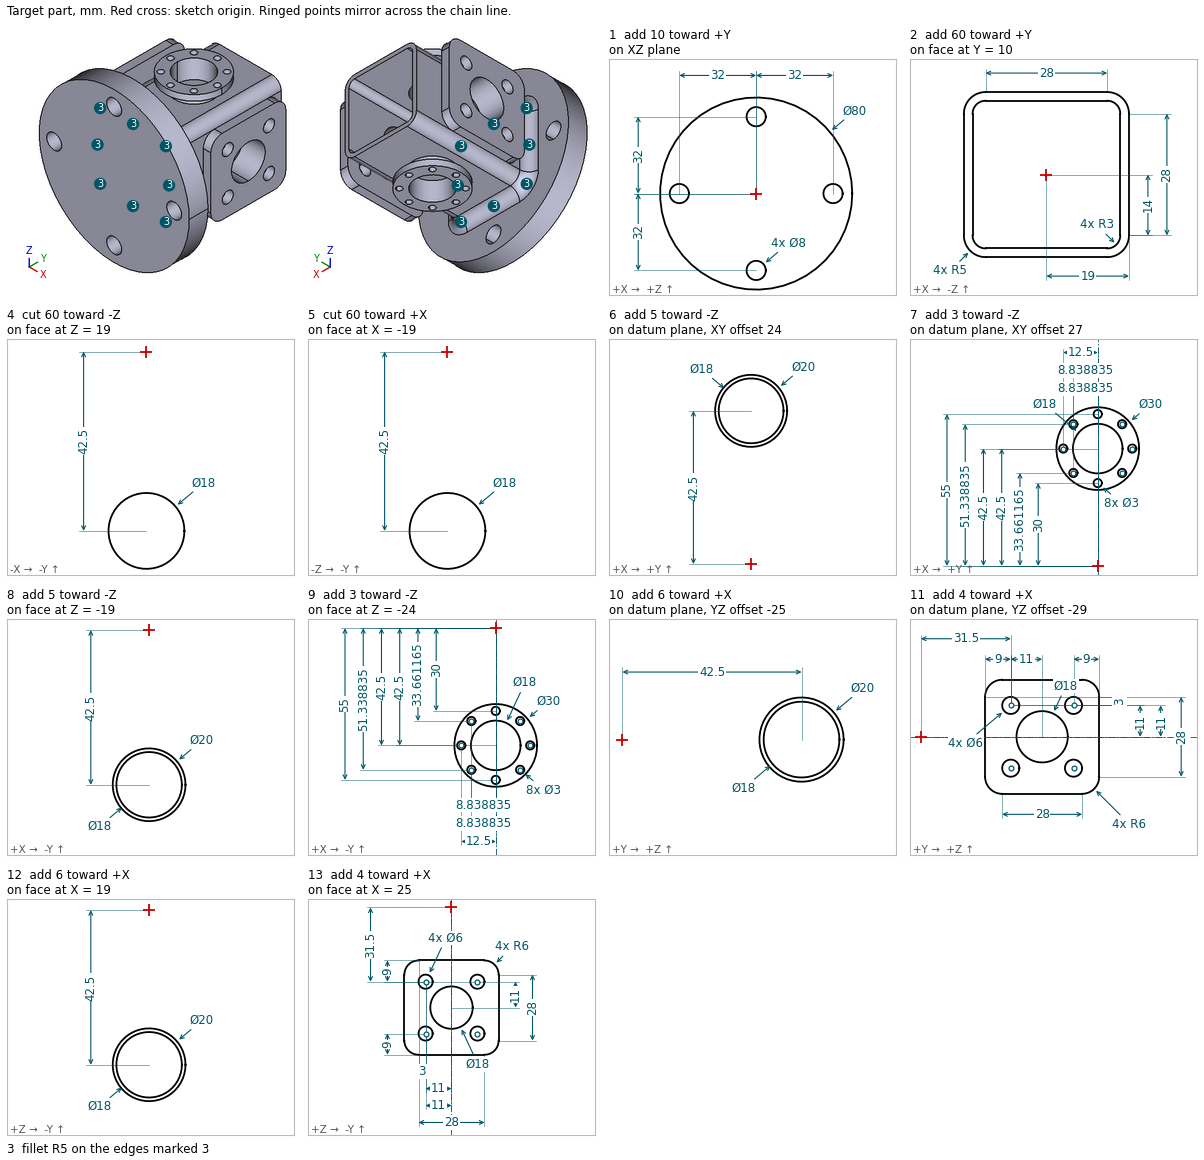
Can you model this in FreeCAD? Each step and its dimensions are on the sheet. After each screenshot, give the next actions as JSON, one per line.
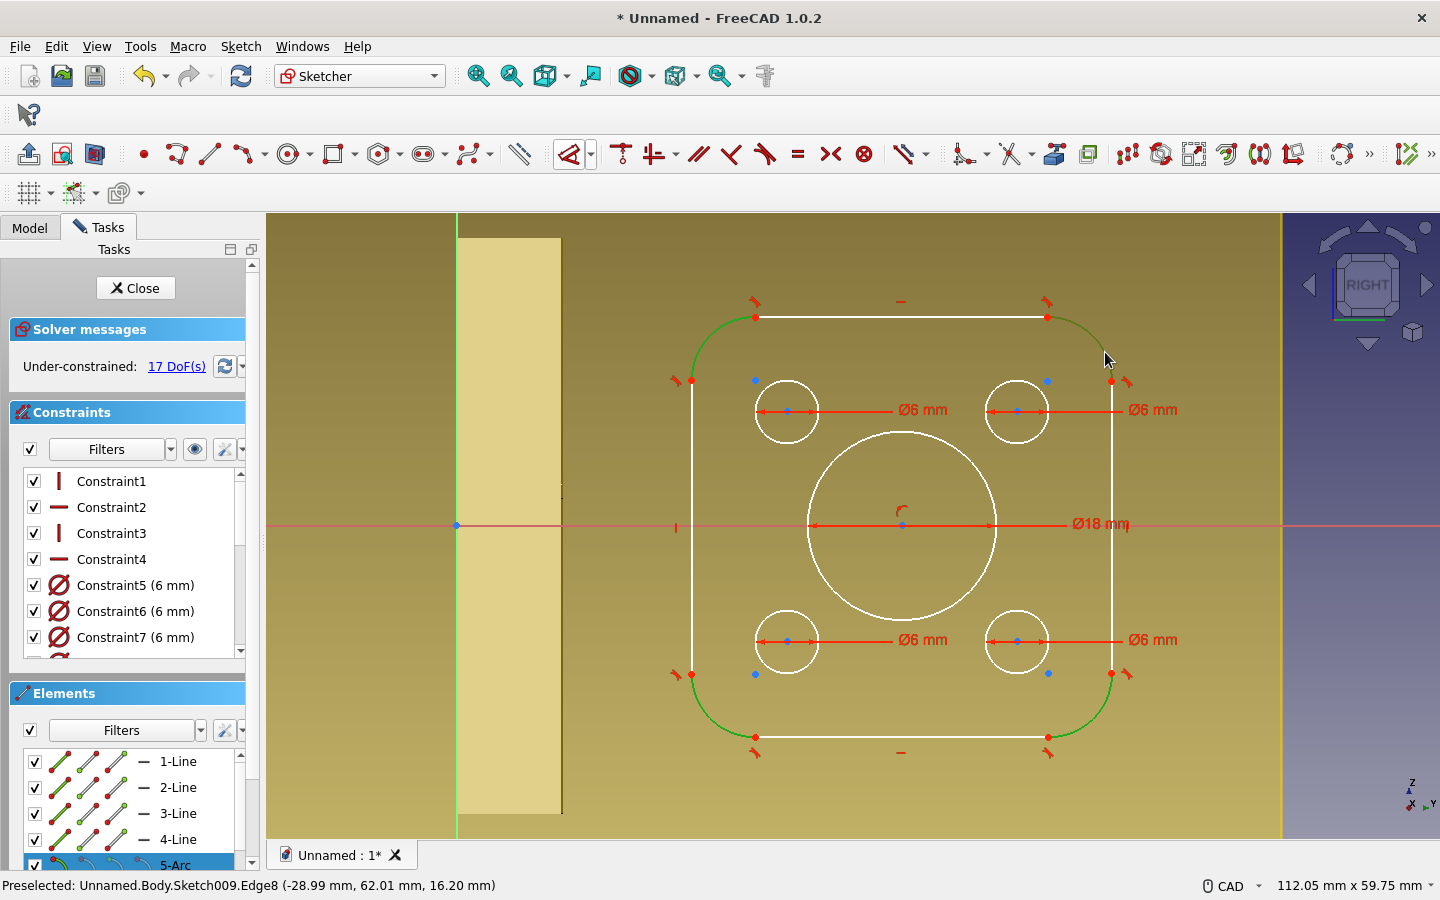
{"action": "left_click", "coordinate": [798, 154]}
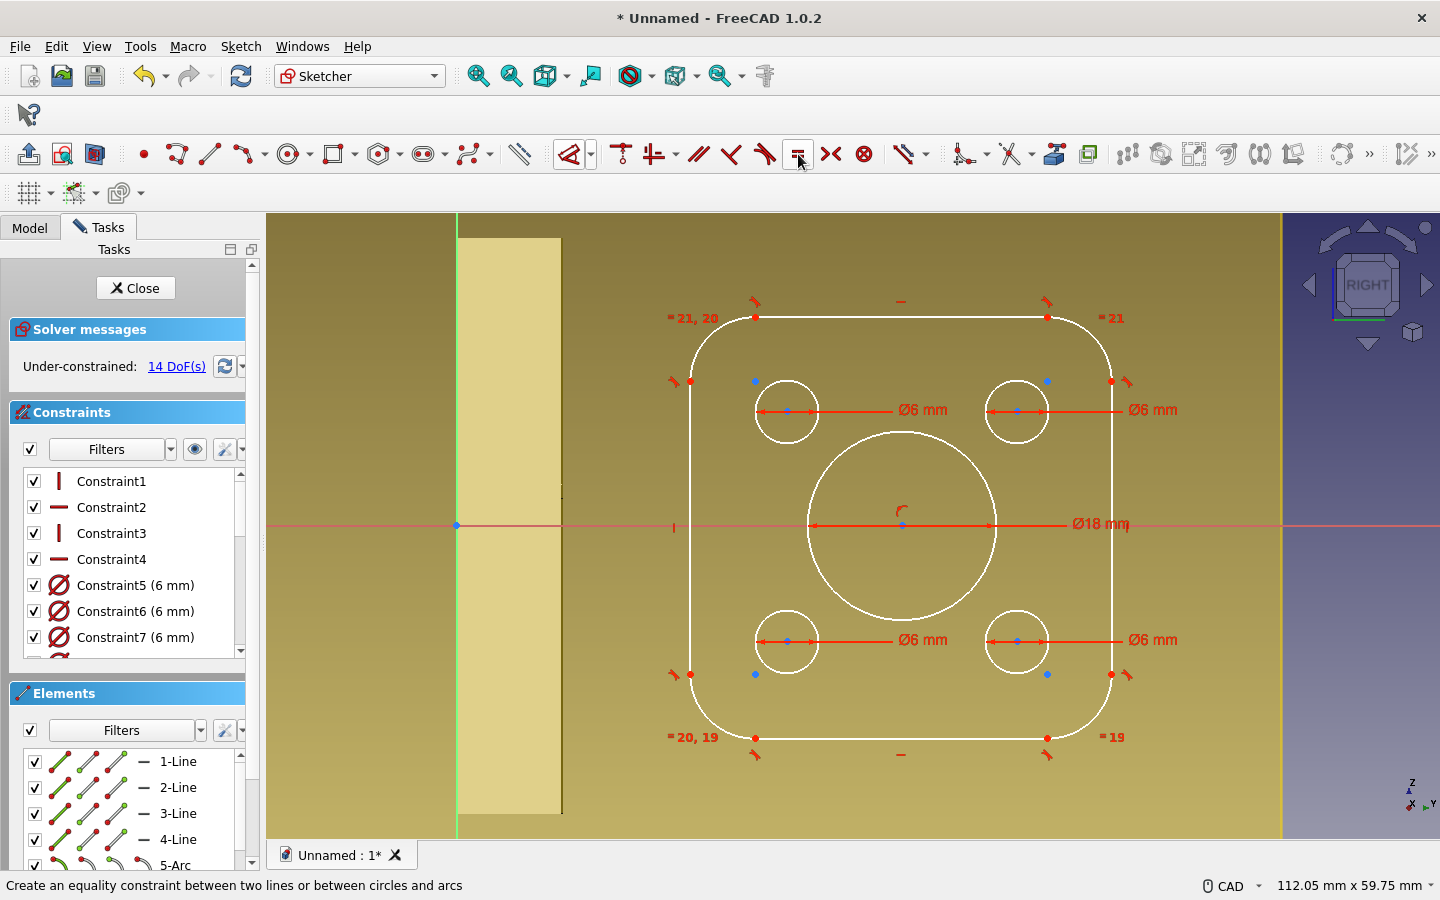
{"action": "left_click", "coordinate": [787, 412]}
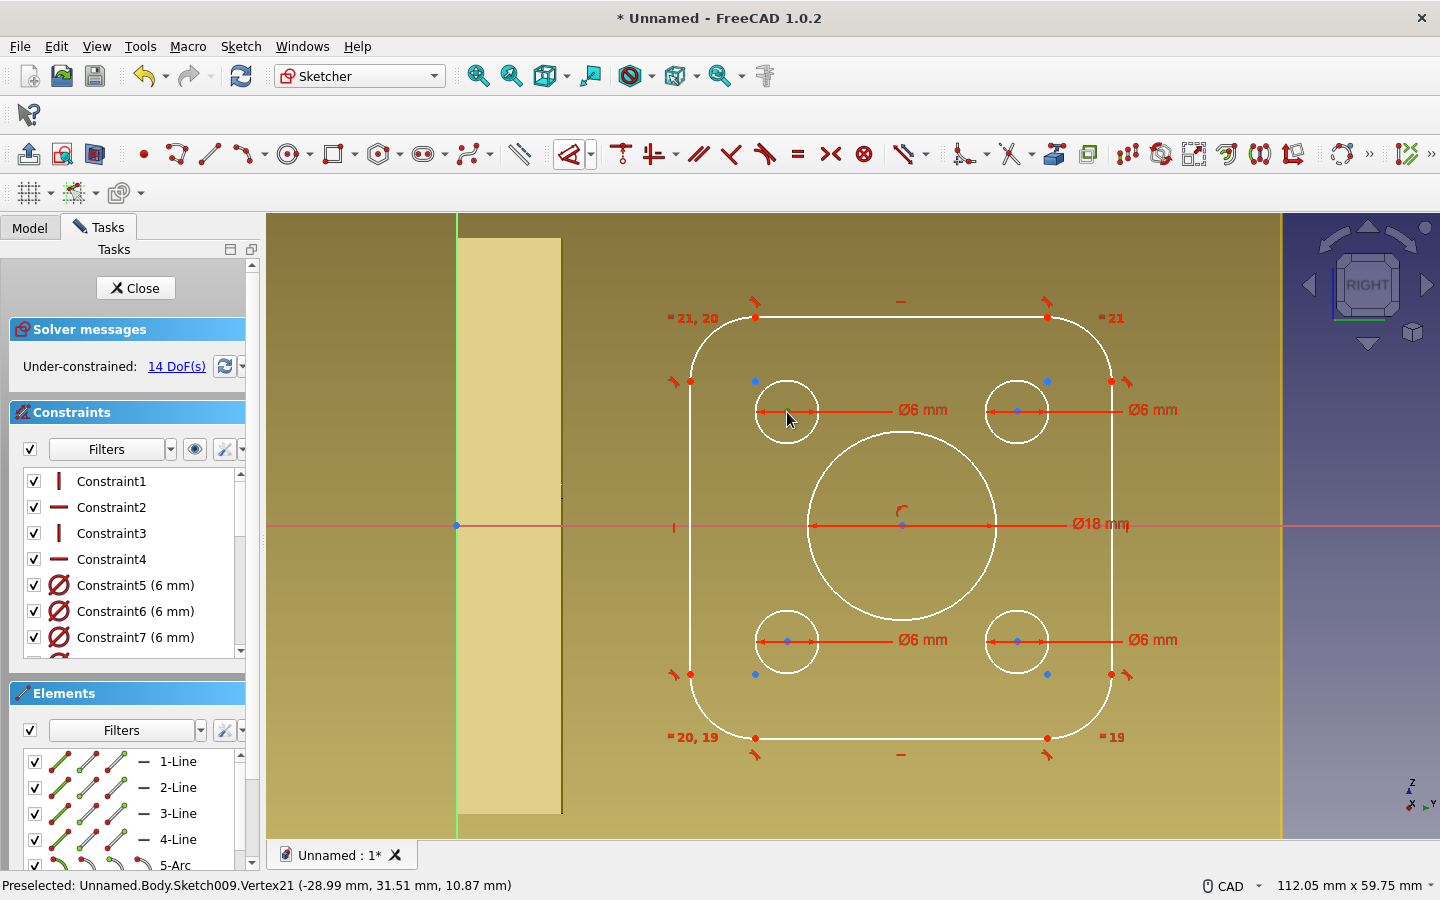
{"action": "left_click", "coordinate": [787, 642]}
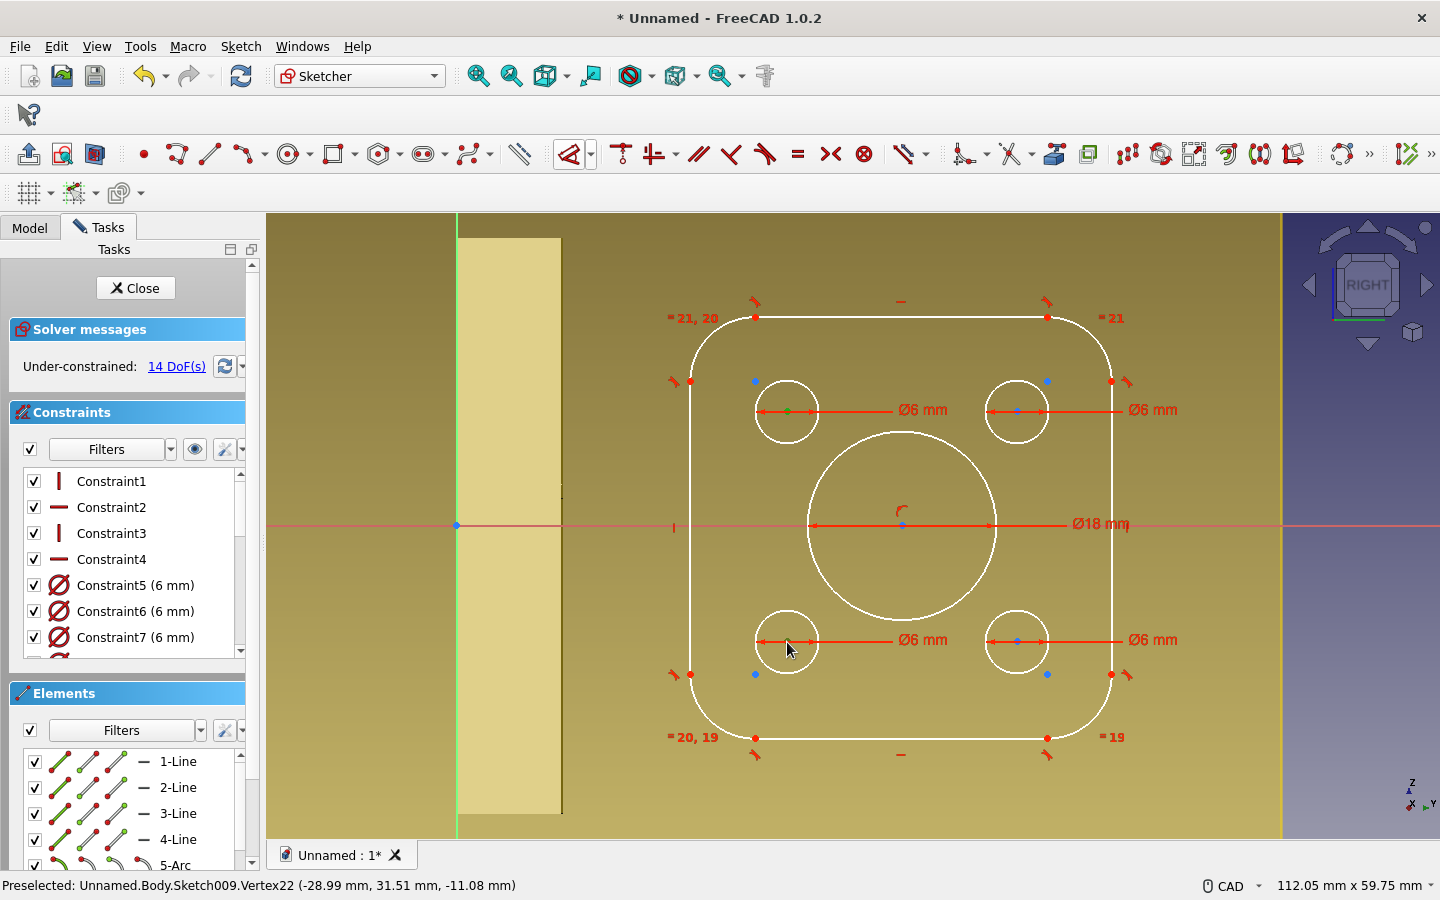
{"action": "left_click", "coordinate": [364, 526]}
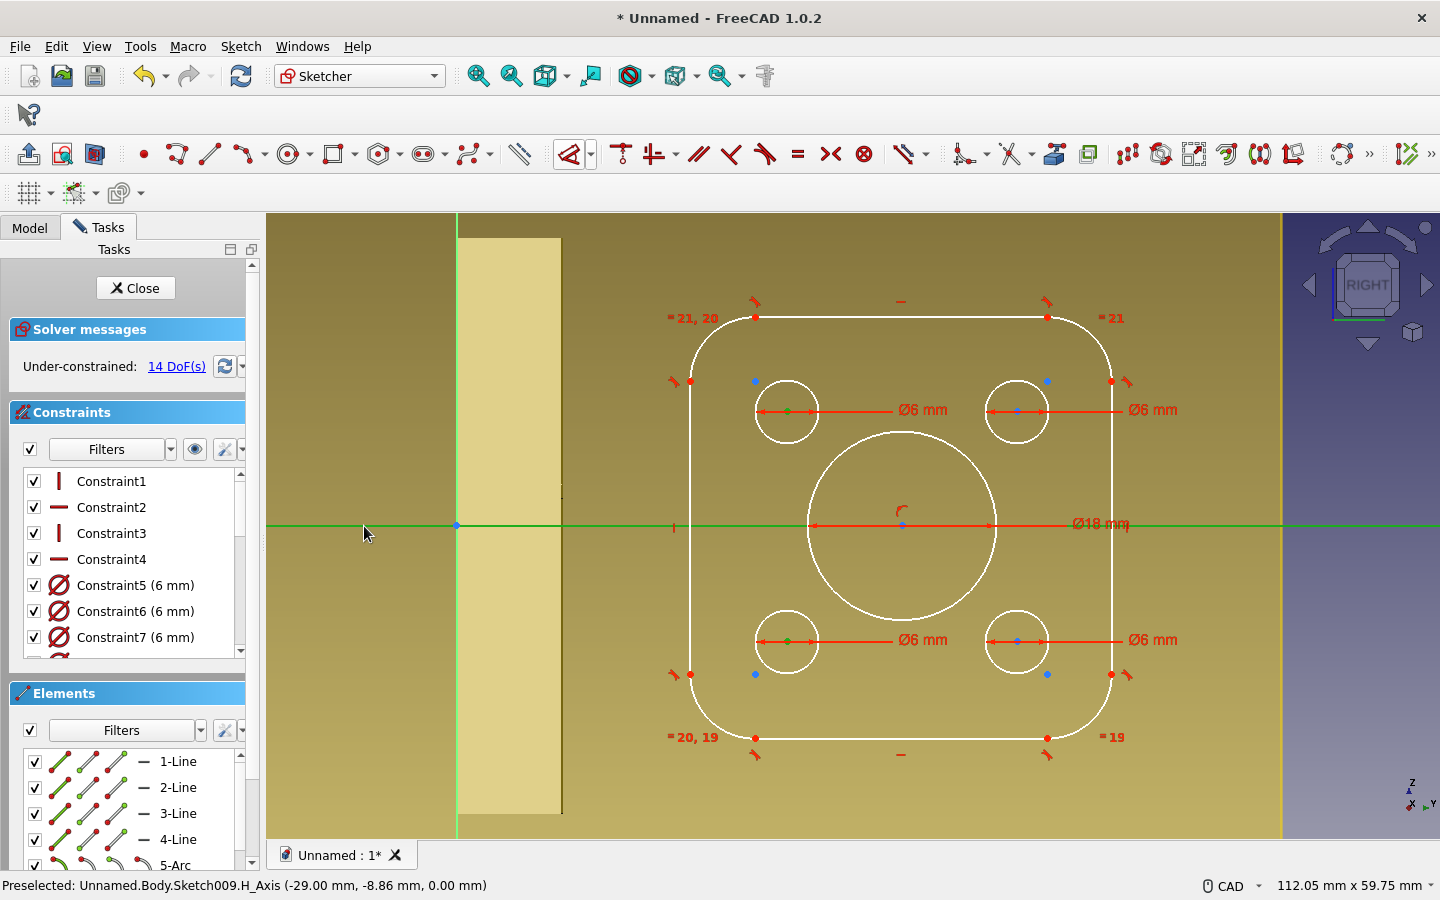
{"action": "key", "text": "s"}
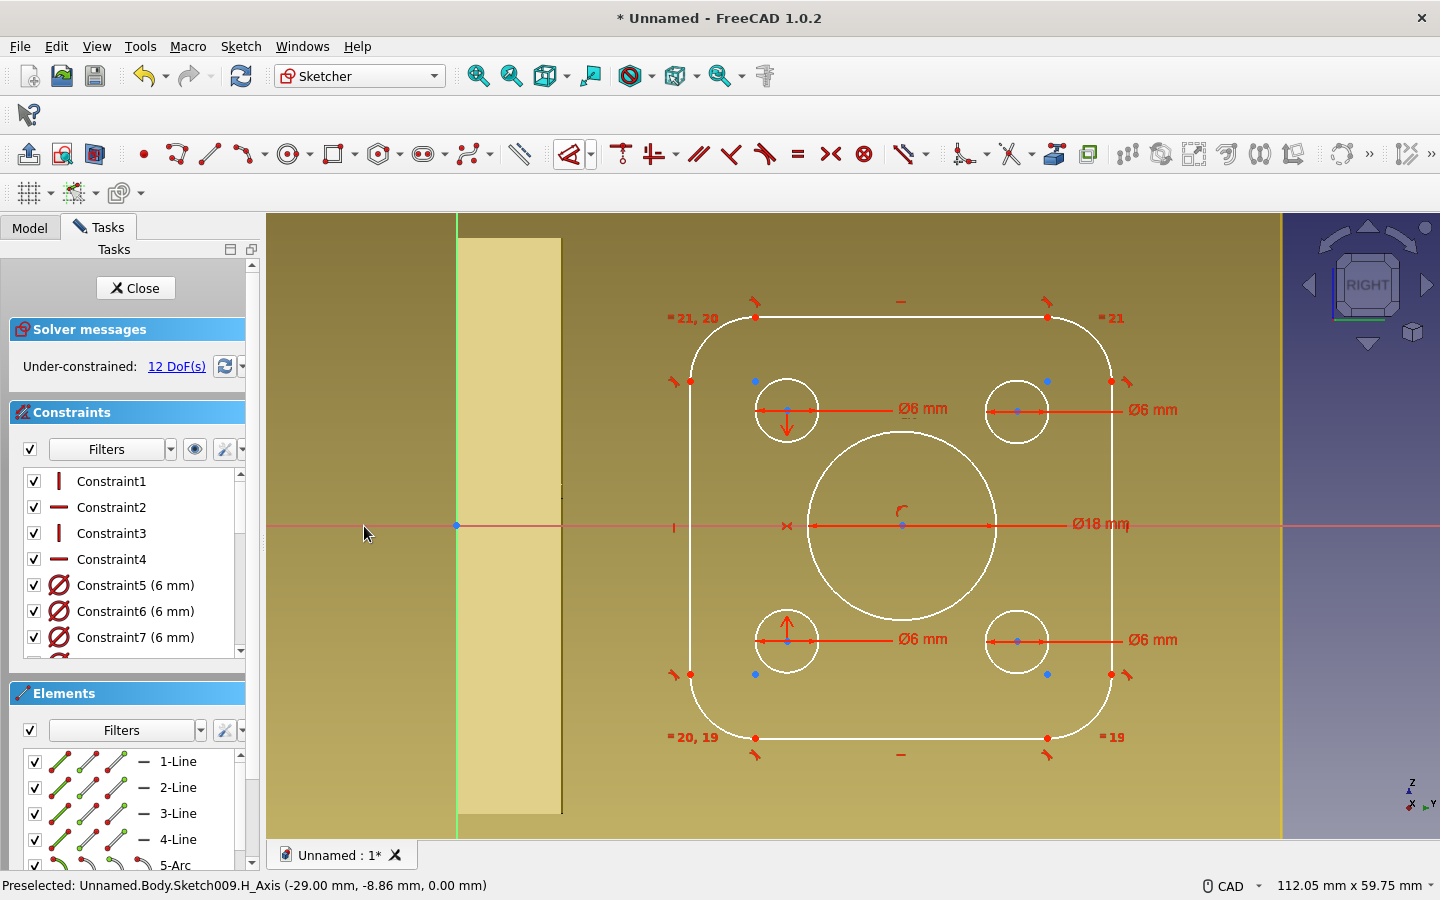
{"action": "left_click", "coordinate": [1017, 412]}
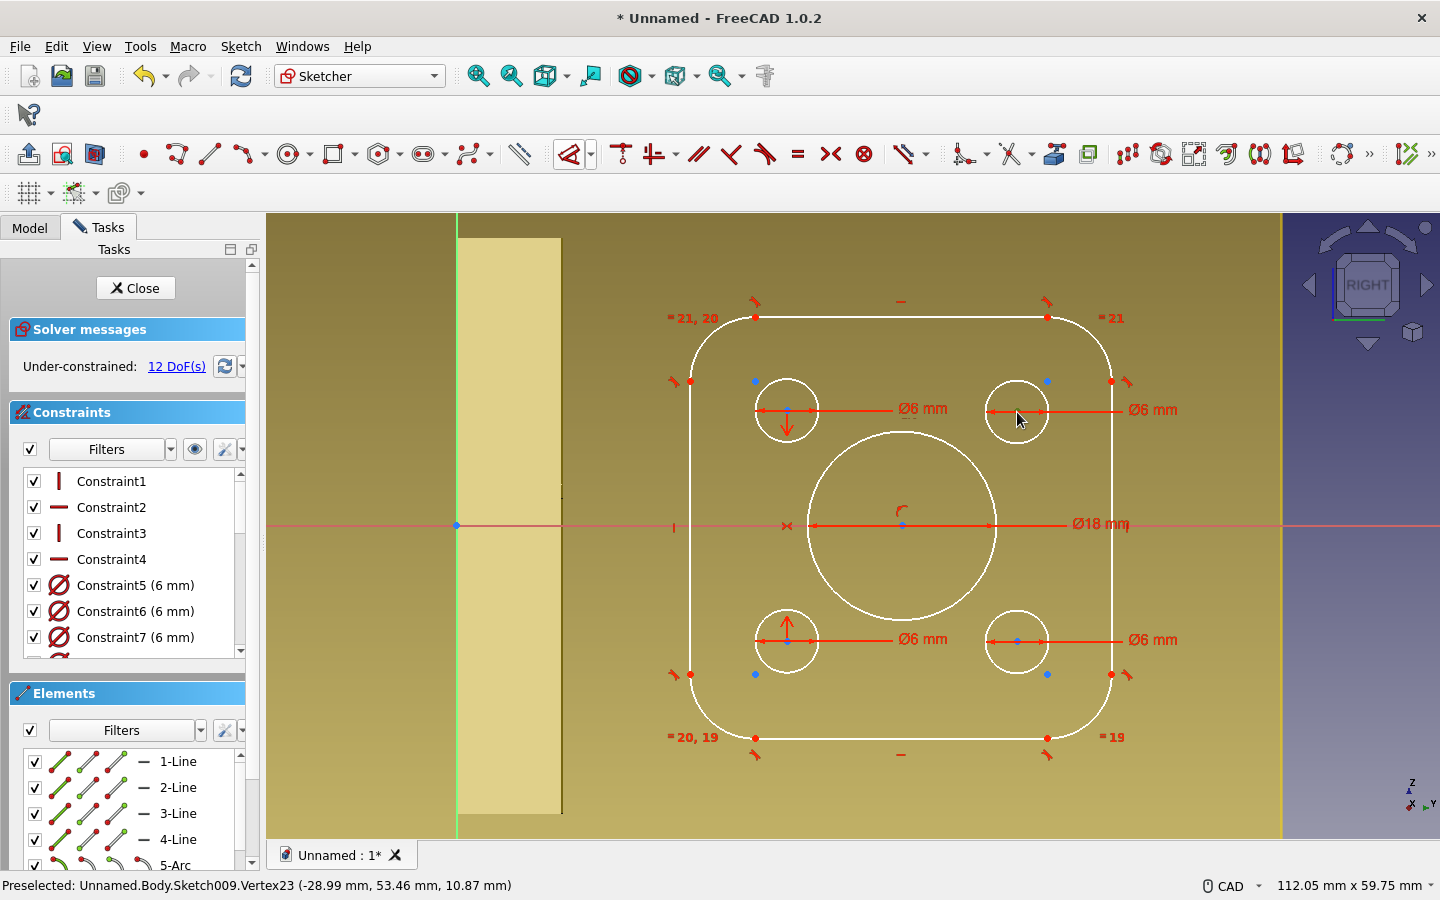
{"action": "left_click", "coordinate": [1017, 642]}